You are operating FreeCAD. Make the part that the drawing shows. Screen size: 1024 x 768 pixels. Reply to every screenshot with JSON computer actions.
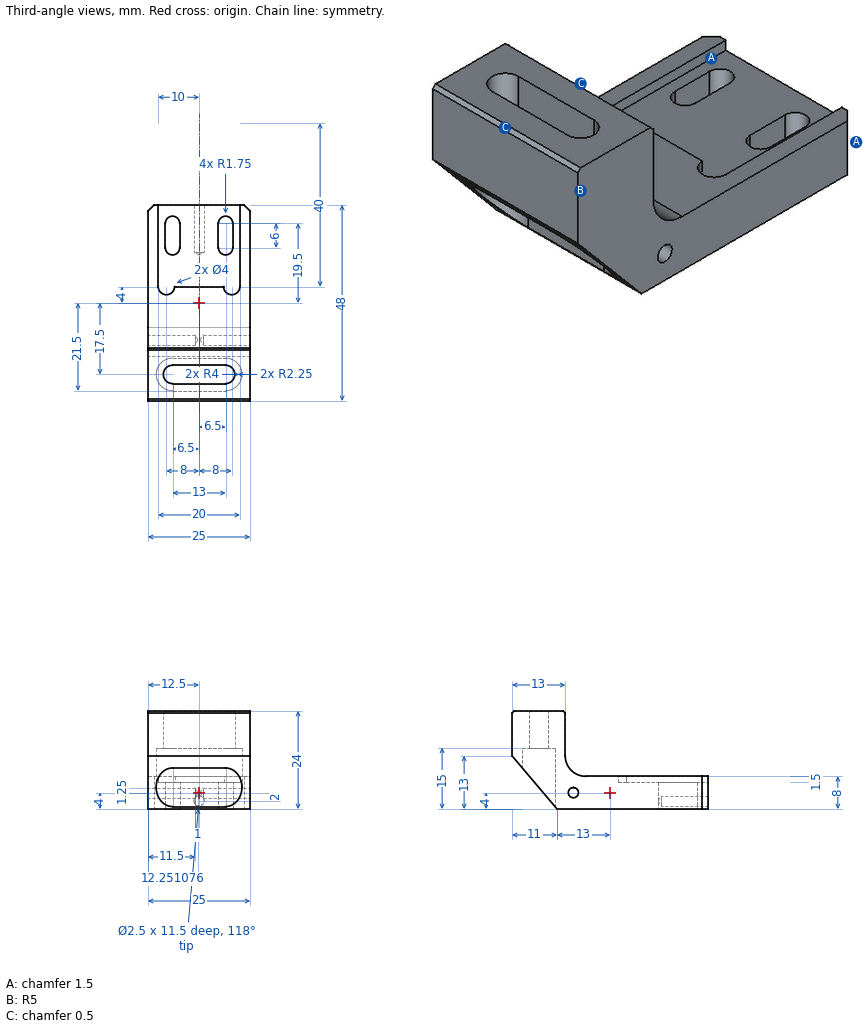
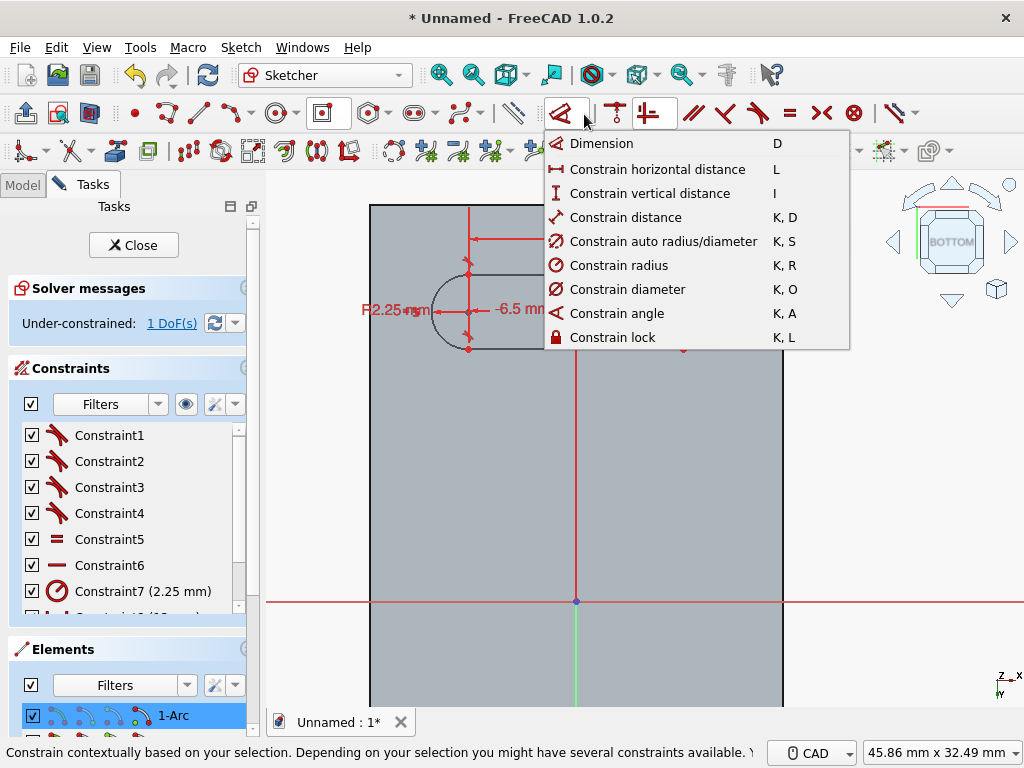
{"action": "left_click", "coordinate": [697, 193]}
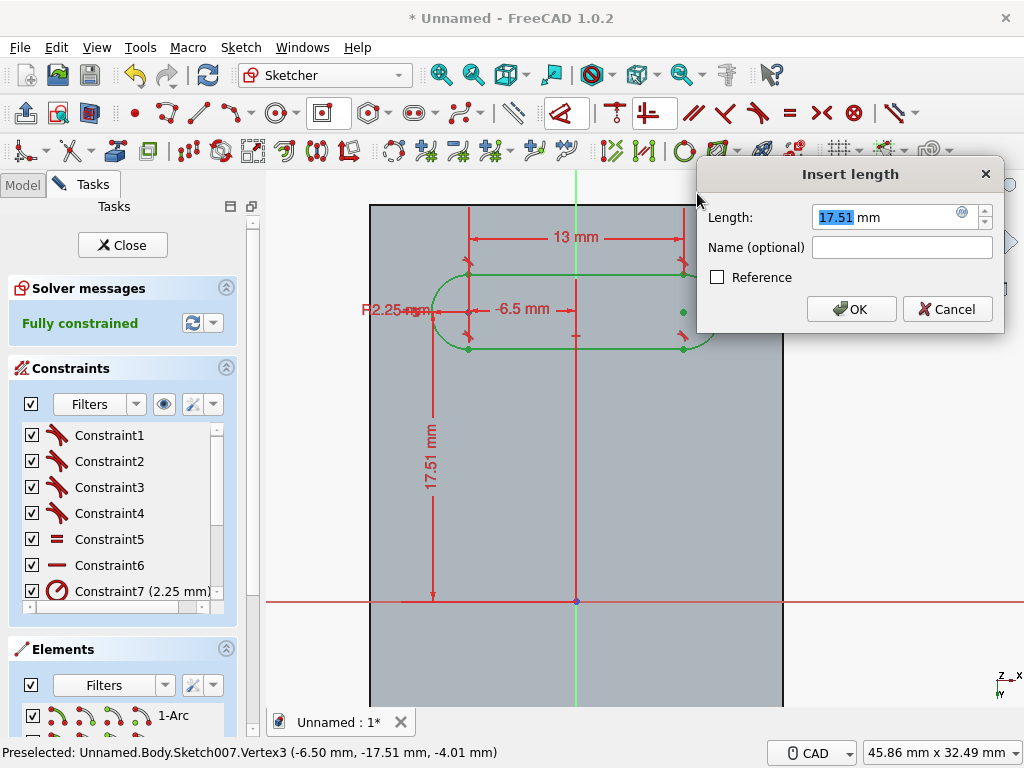
{"action": "type", "text": "17.5"}
{"action": "key", "text": "Return"}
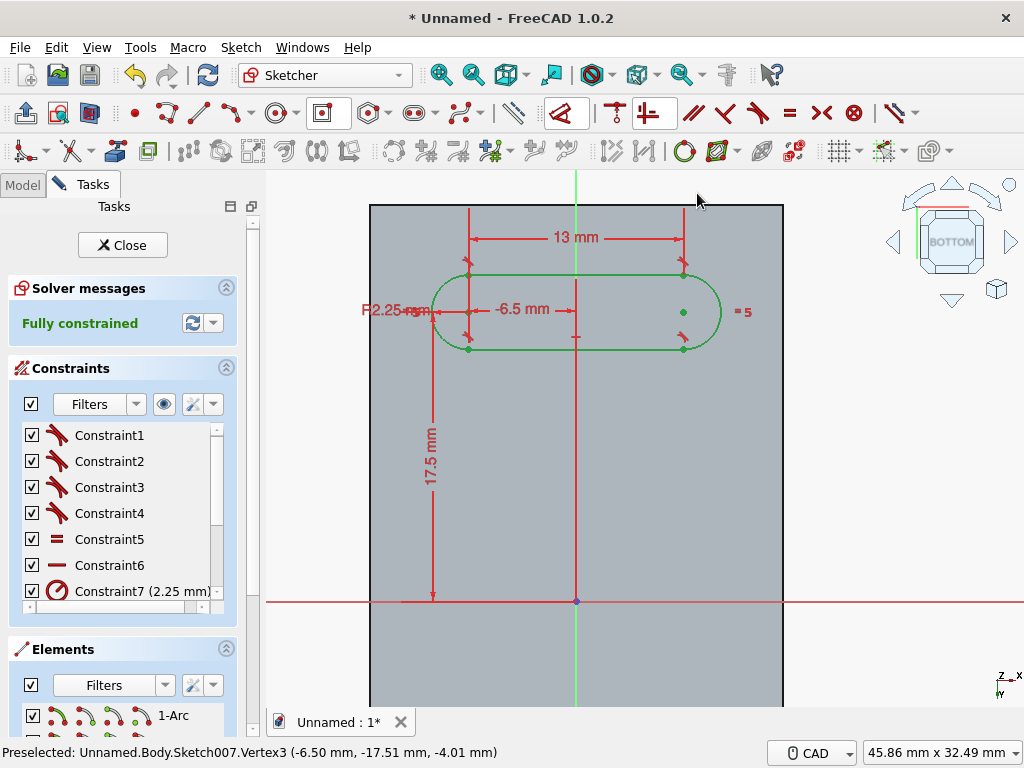
{"action": "left_click", "coordinate": [123, 245]}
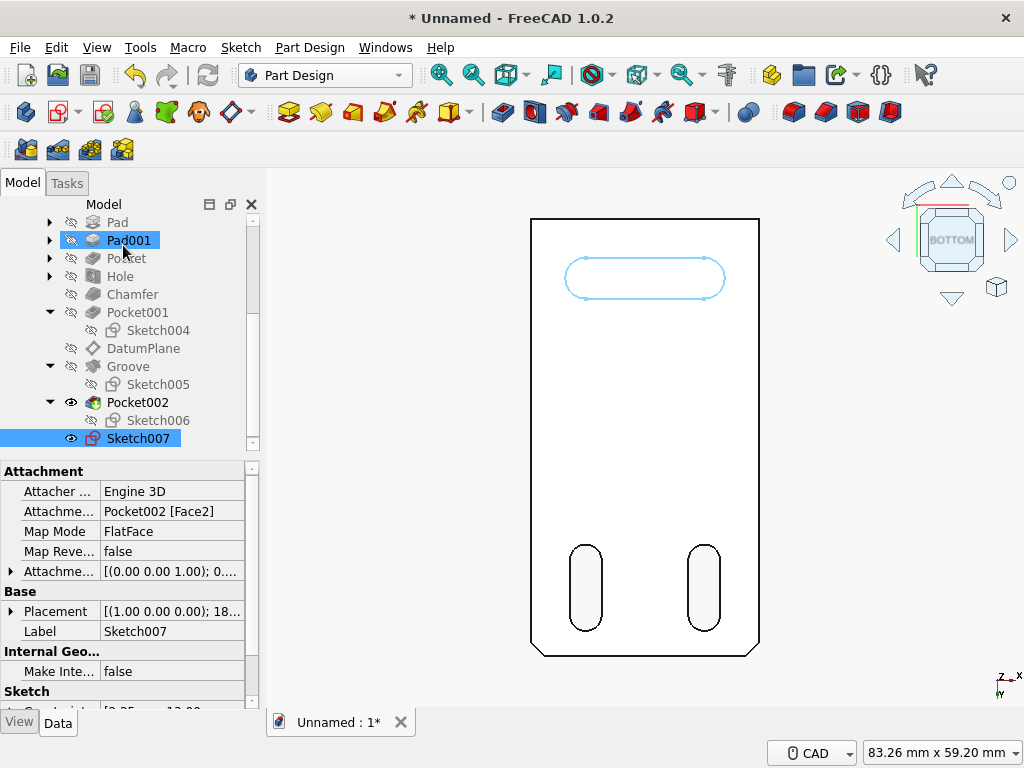
{"action": "left_click", "coordinate": [504, 112]}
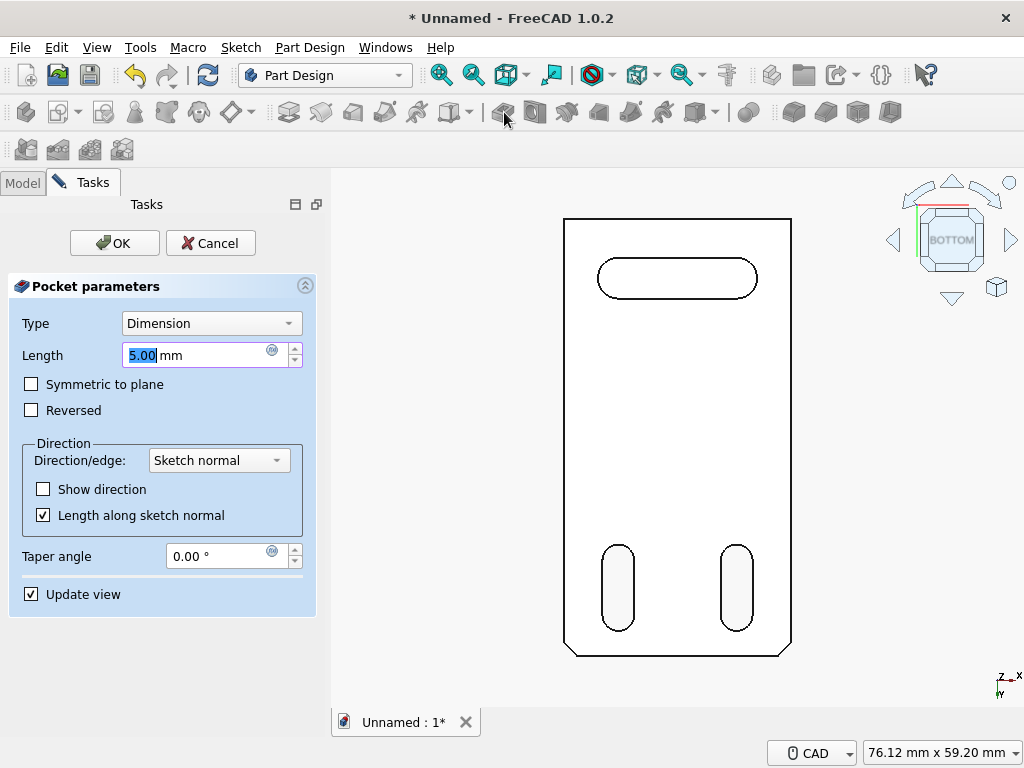
{"action": "left_click", "coordinate": [212, 324]}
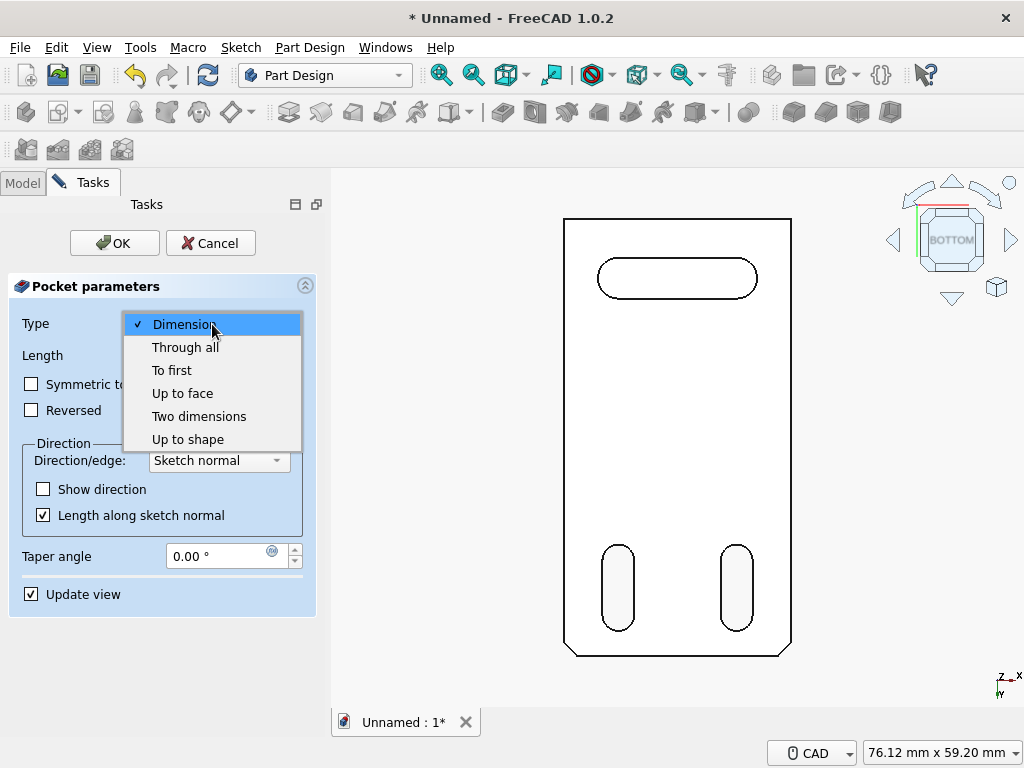
{"action": "left_click", "coordinate": [212, 348]}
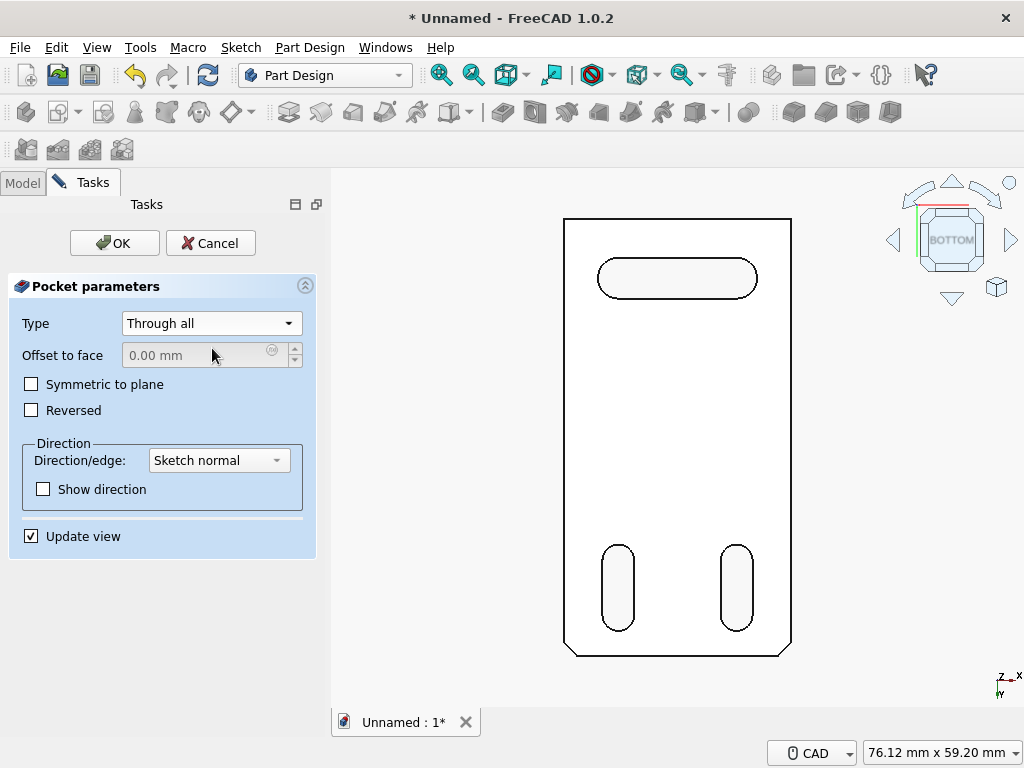
{"action": "left_click", "coordinate": [115, 243]}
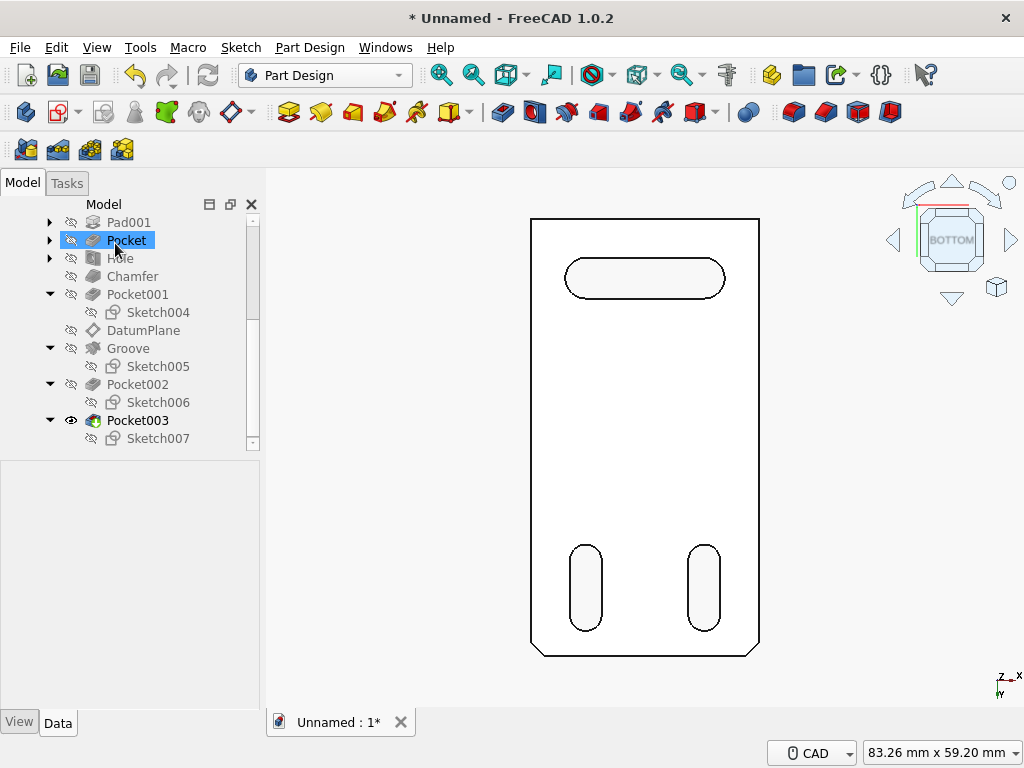
{"action": "key", "text": "0"}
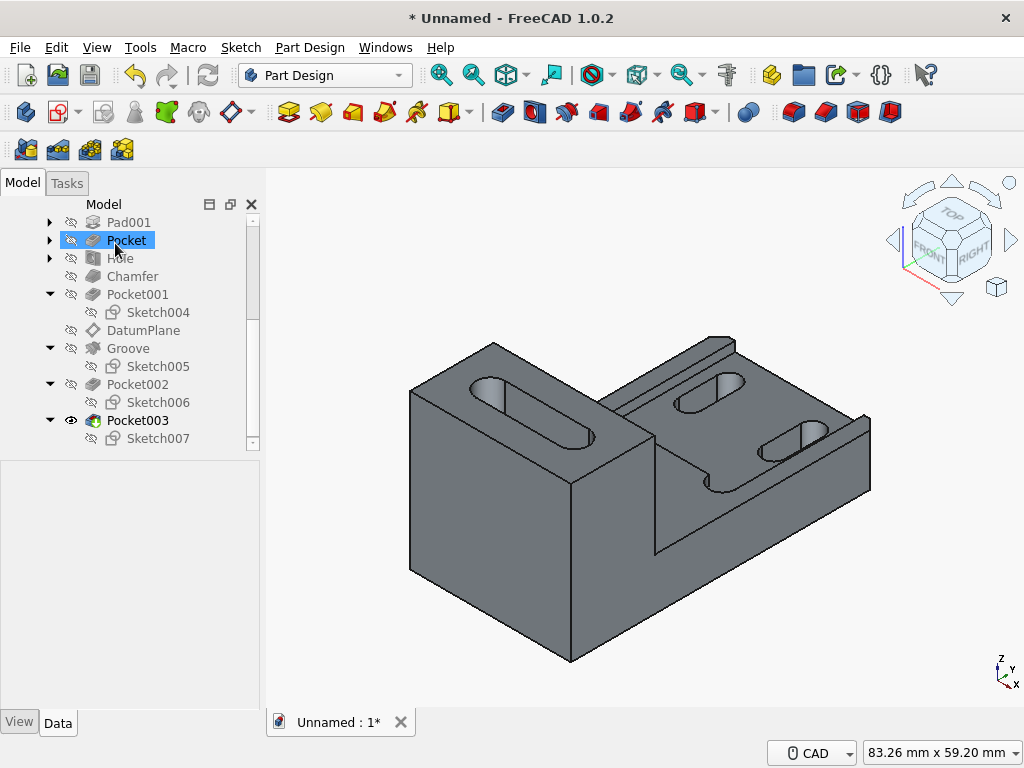
{"action": "left_click", "coordinate": [635, 586]}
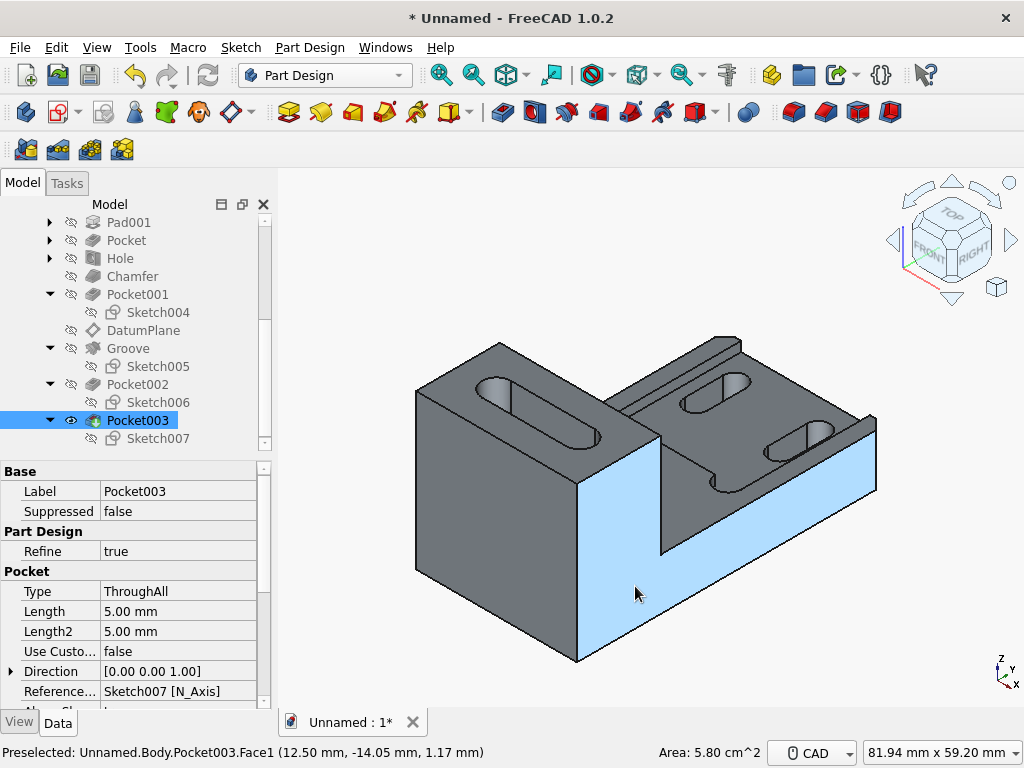
{"action": "left_click", "coordinate": [58, 112]}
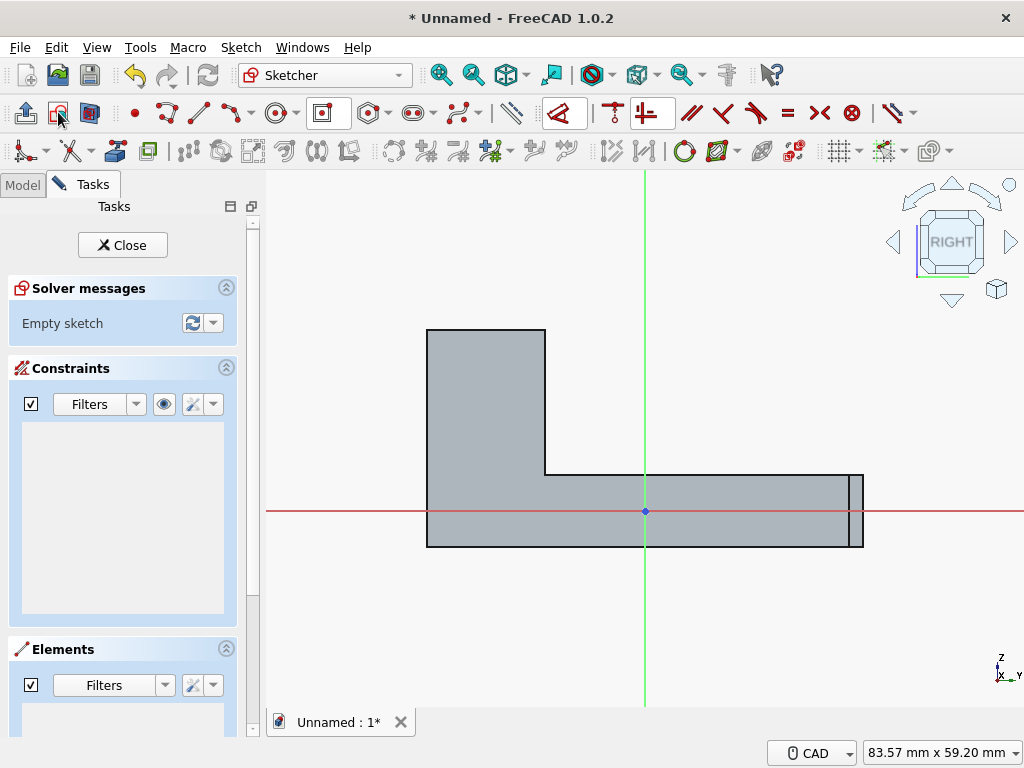
{"action": "scroll", "coordinate": [487, 549], "scroll_direction": "up", "scroll_amount": 3}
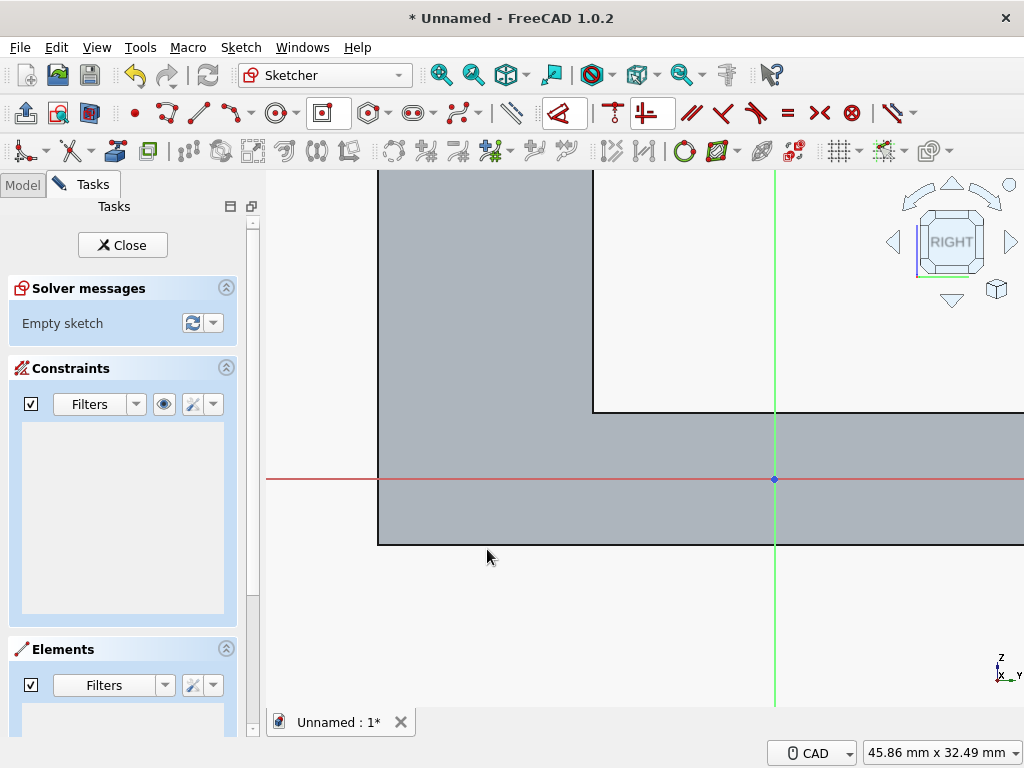
{"action": "left_click", "coordinate": [168, 114]}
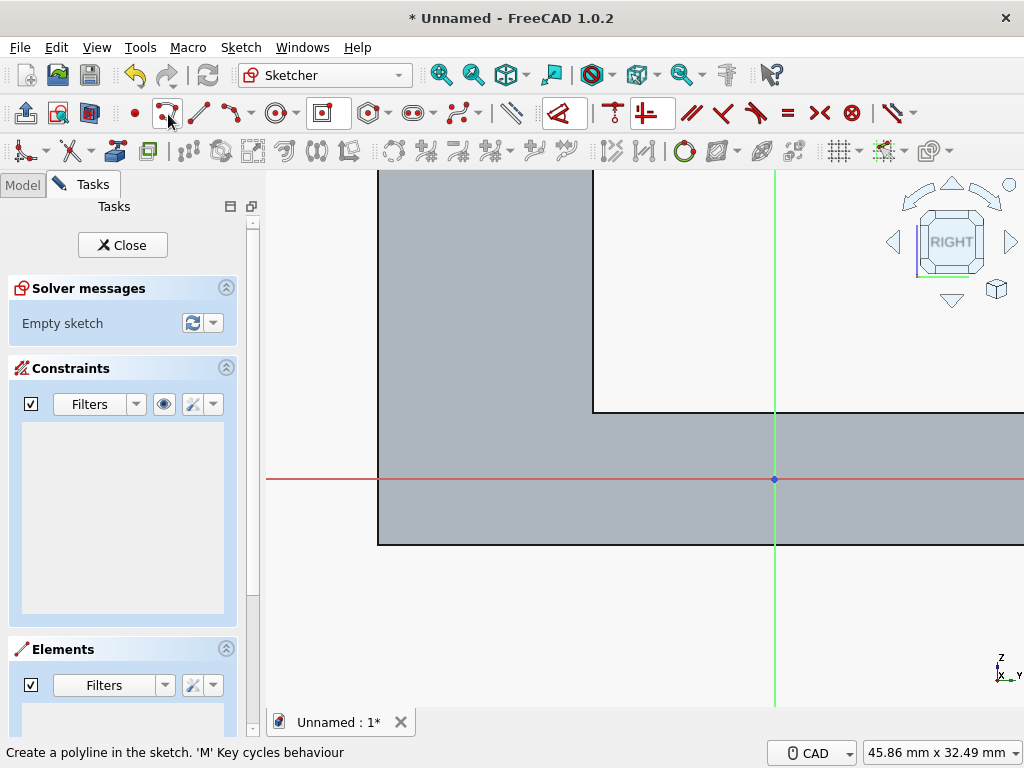
{"action": "left_click", "coordinate": [560, 545]}
{"action": "left_click", "coordinate": [378, 331]}
{"action": "left_click", "coordinate": [378, 545]}
{"action": "left_click", "coordinate": [560, 546]}
{"action": "key", "text": "Escape"}
{"action": "key", "text": "Escape"}